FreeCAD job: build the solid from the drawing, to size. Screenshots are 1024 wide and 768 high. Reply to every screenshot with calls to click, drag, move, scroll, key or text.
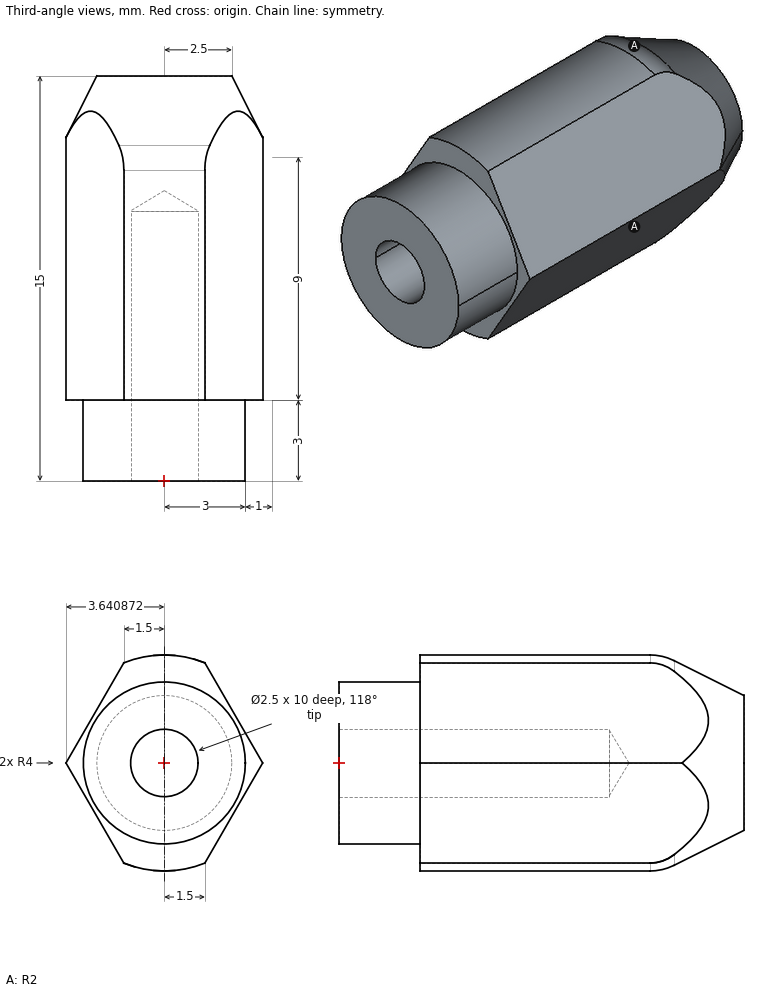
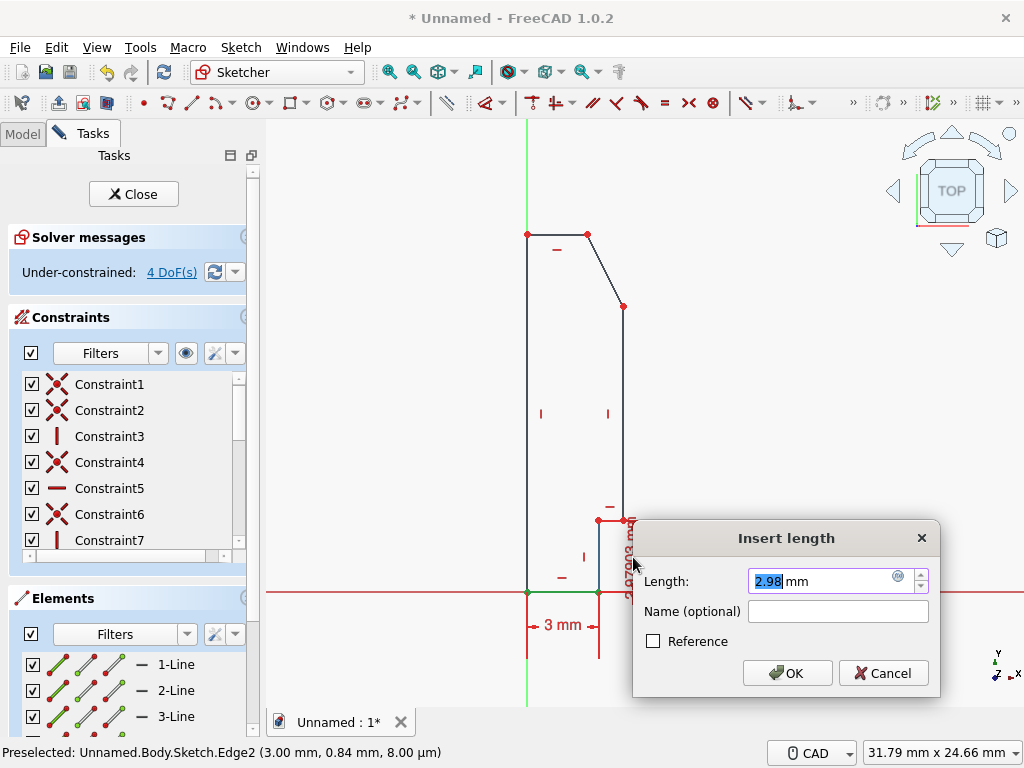
text(3)
key(Return)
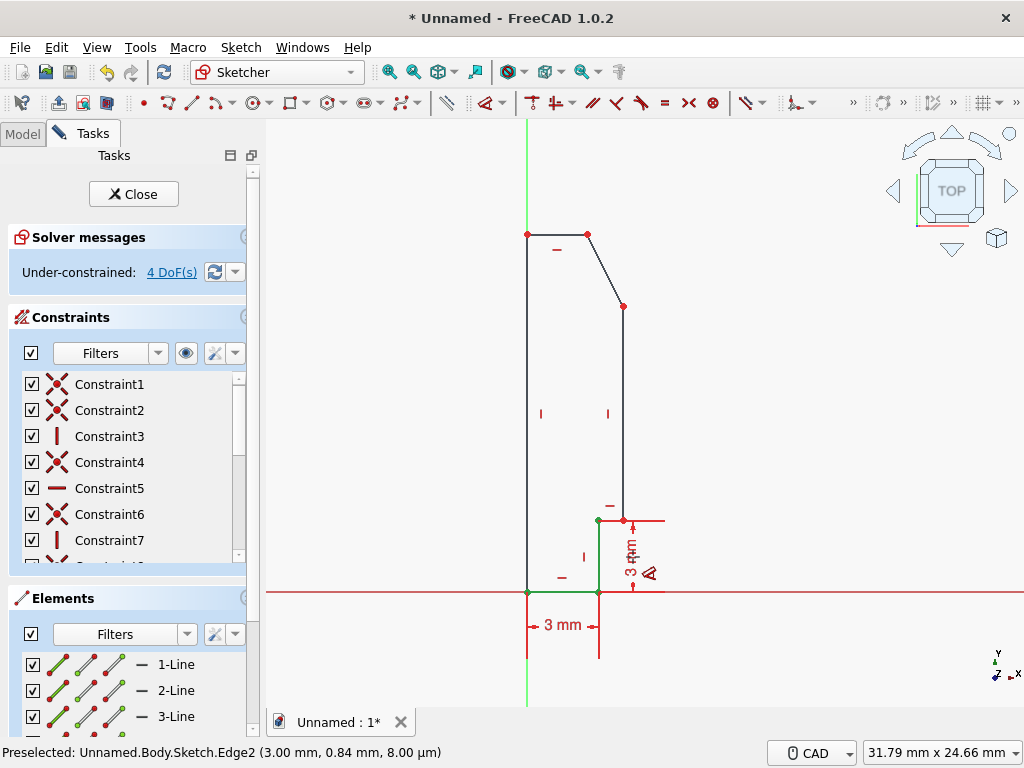
scroll(608, 520, up, 3)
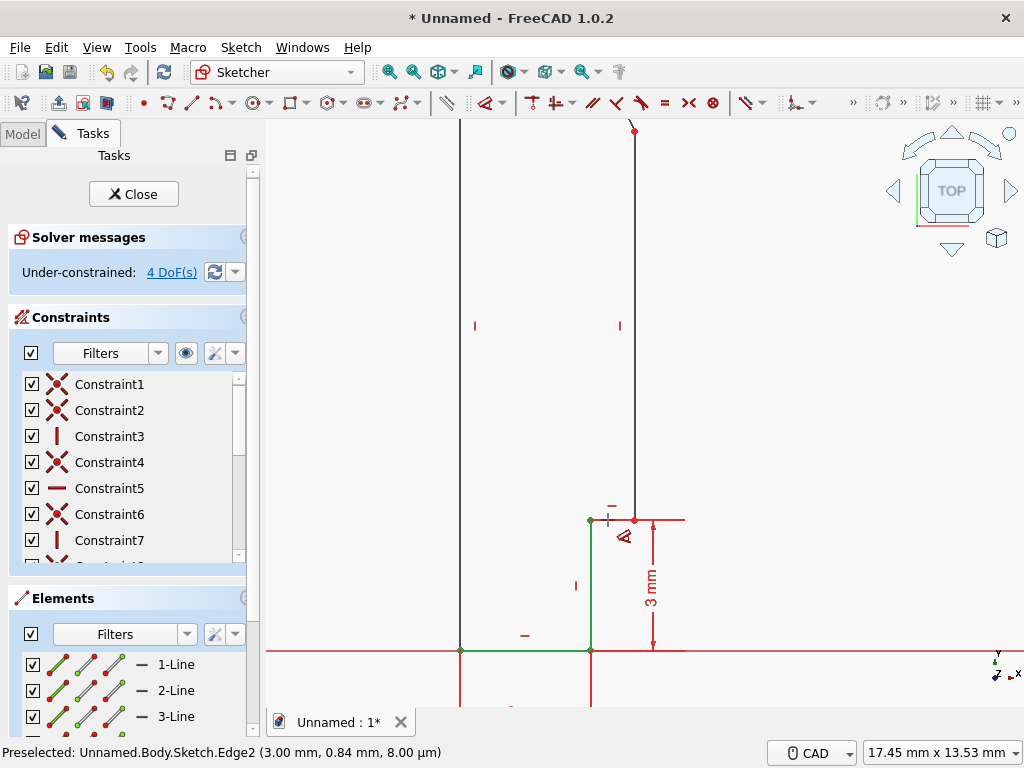
click(608, 520)
click(613, 554)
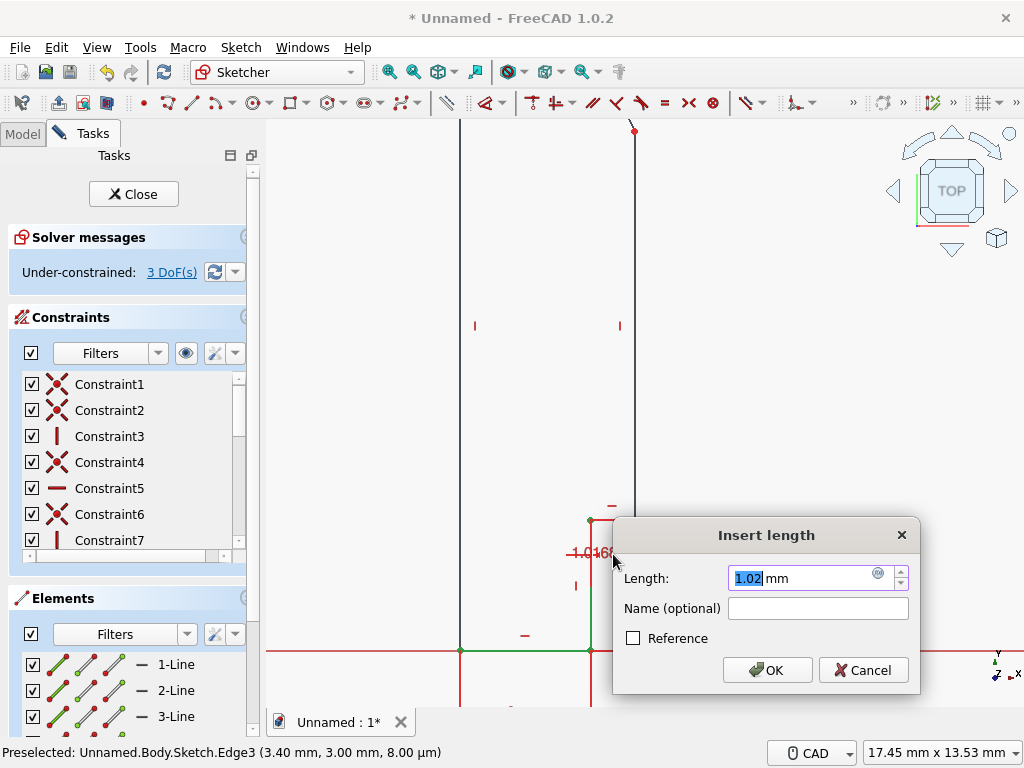
text(1)
key(Return)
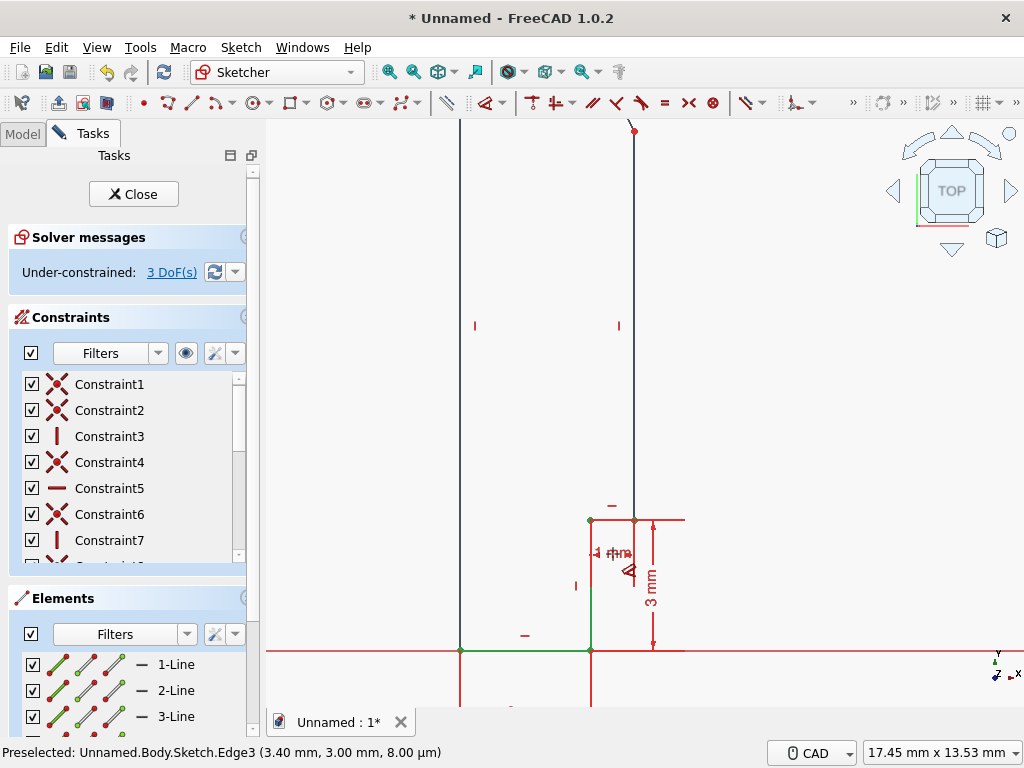
click(634, 404)
click(668, 334)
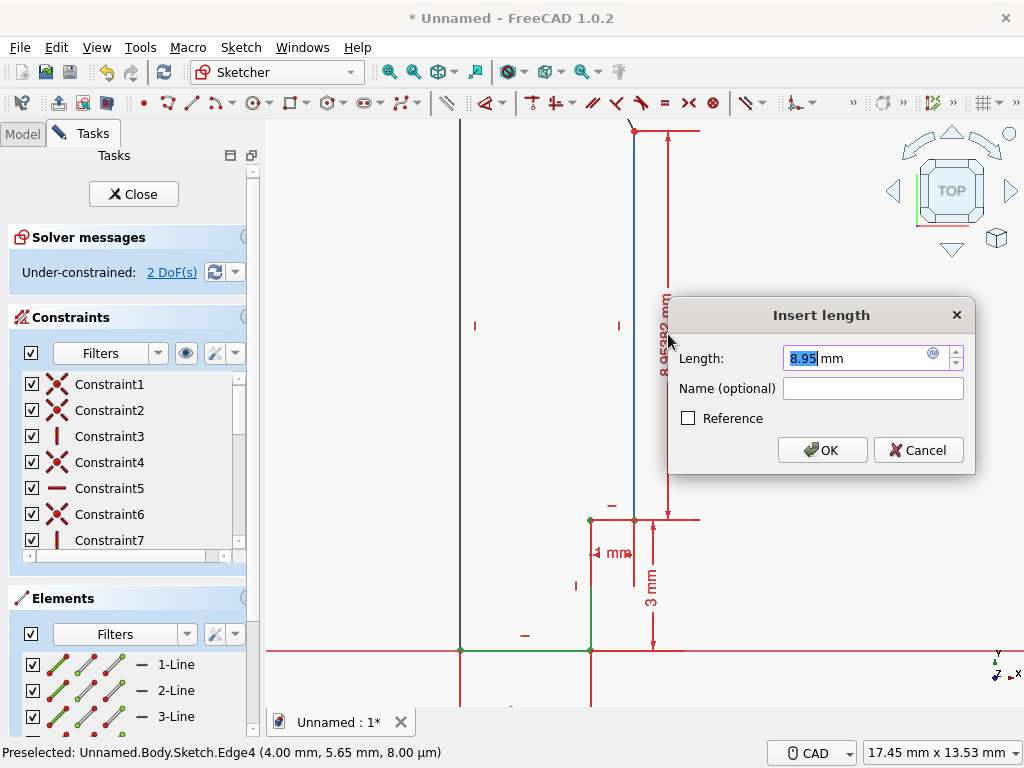
text(9)
key(Return)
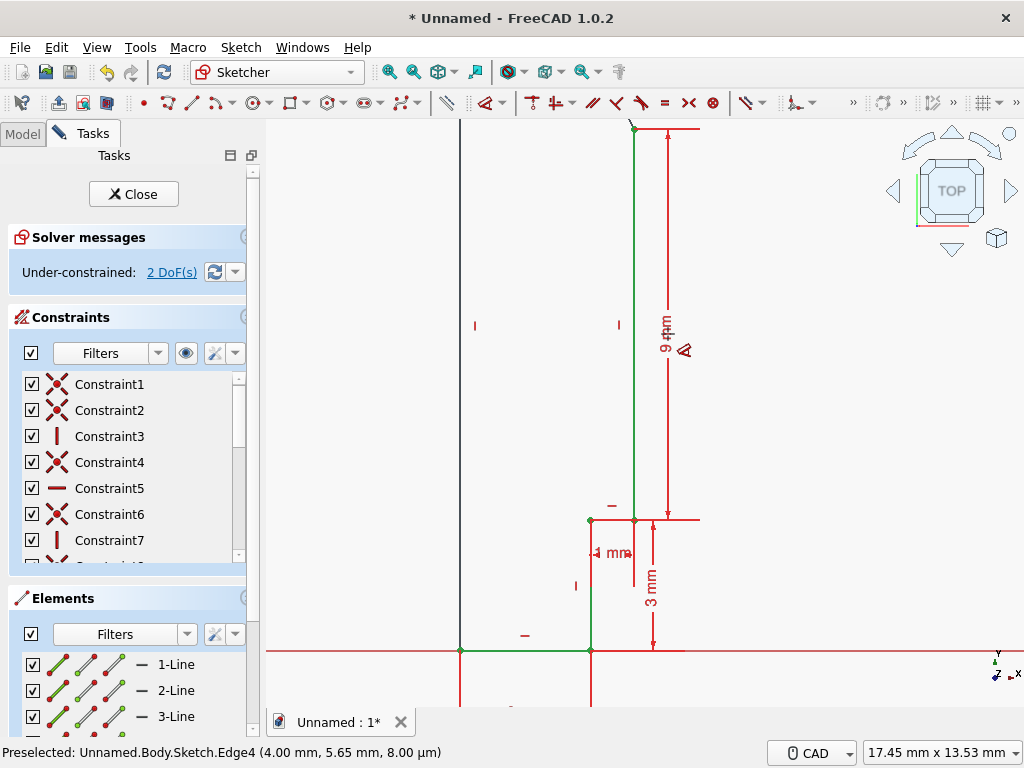
click(460, 195)
click(426, 399)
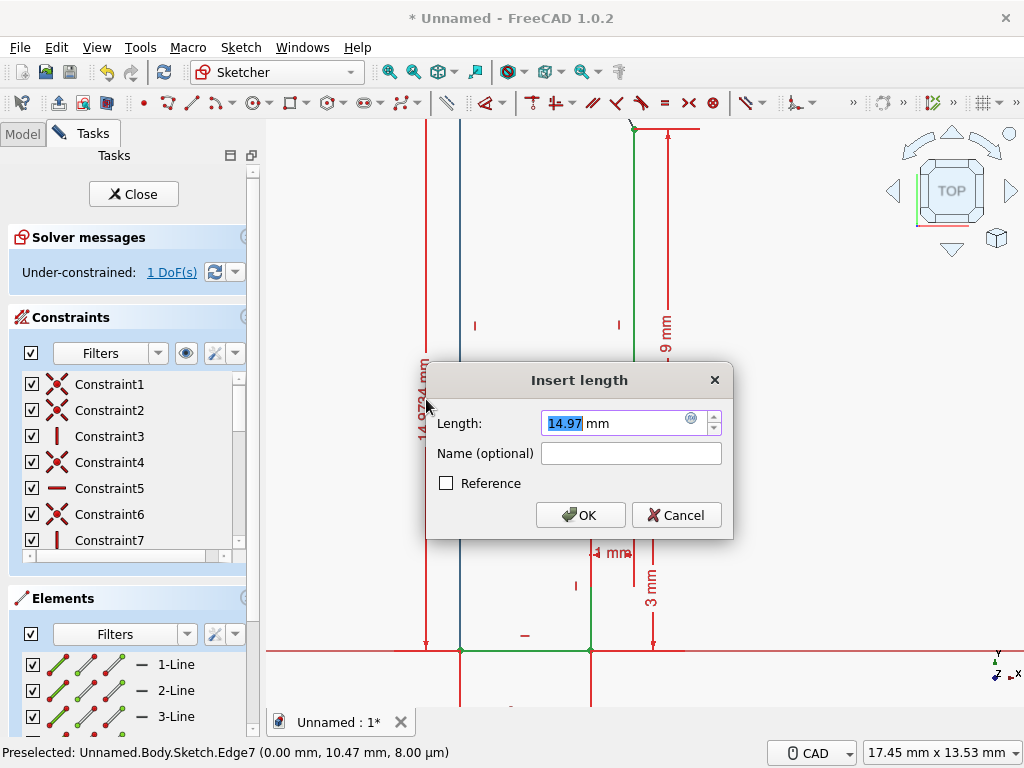
text(15)
key(Return)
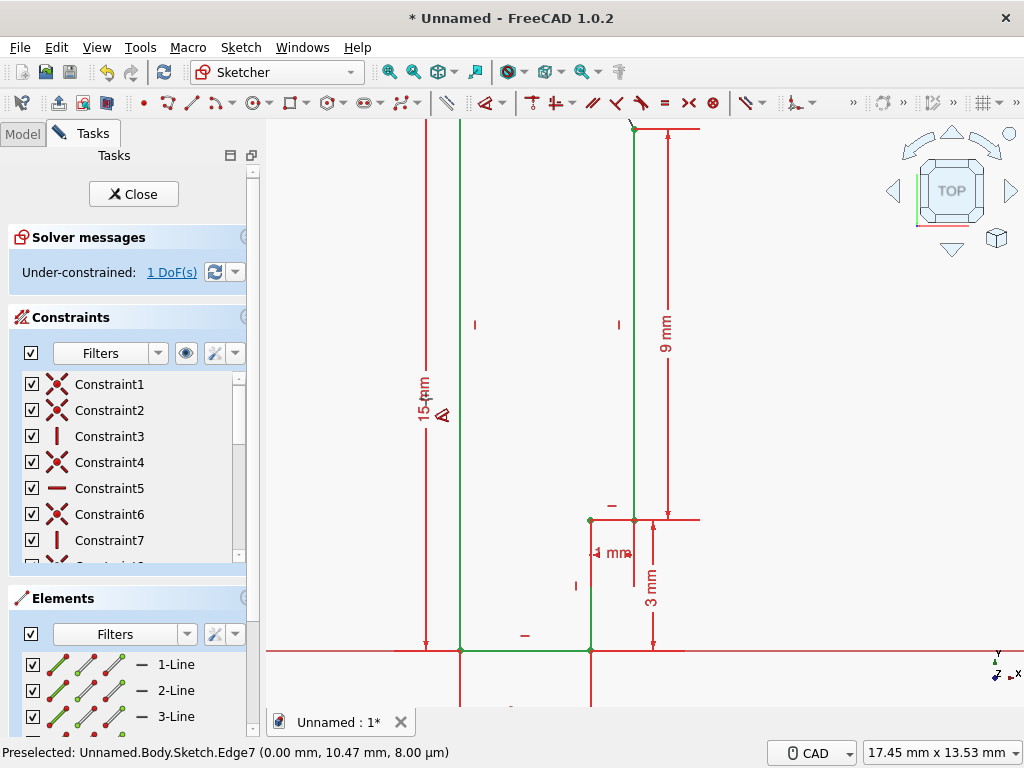
scroll(612, 520, down, 3)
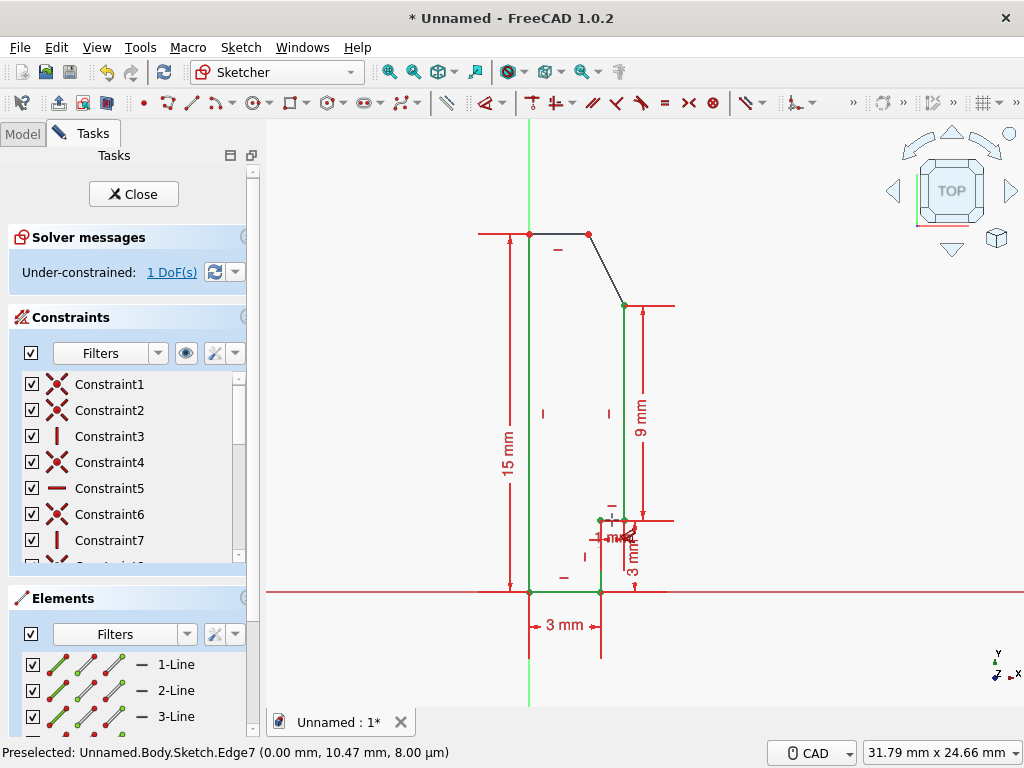
click(571, 234)
click(559, 200)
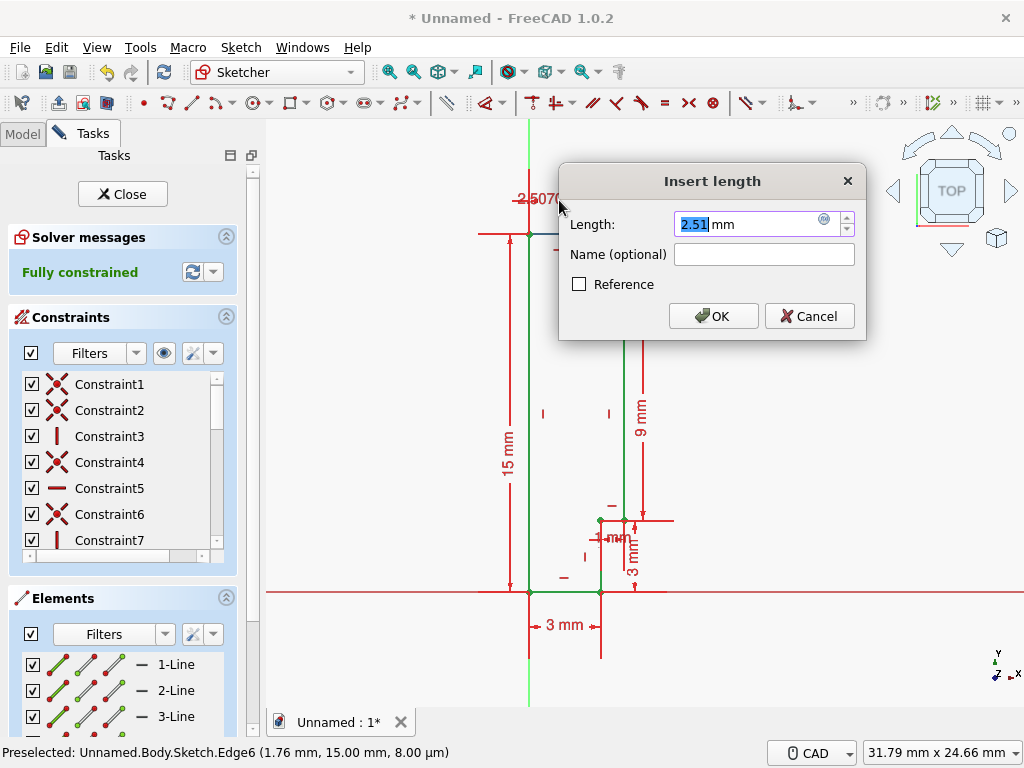
text(2.5)
key(Return)
key(Escape)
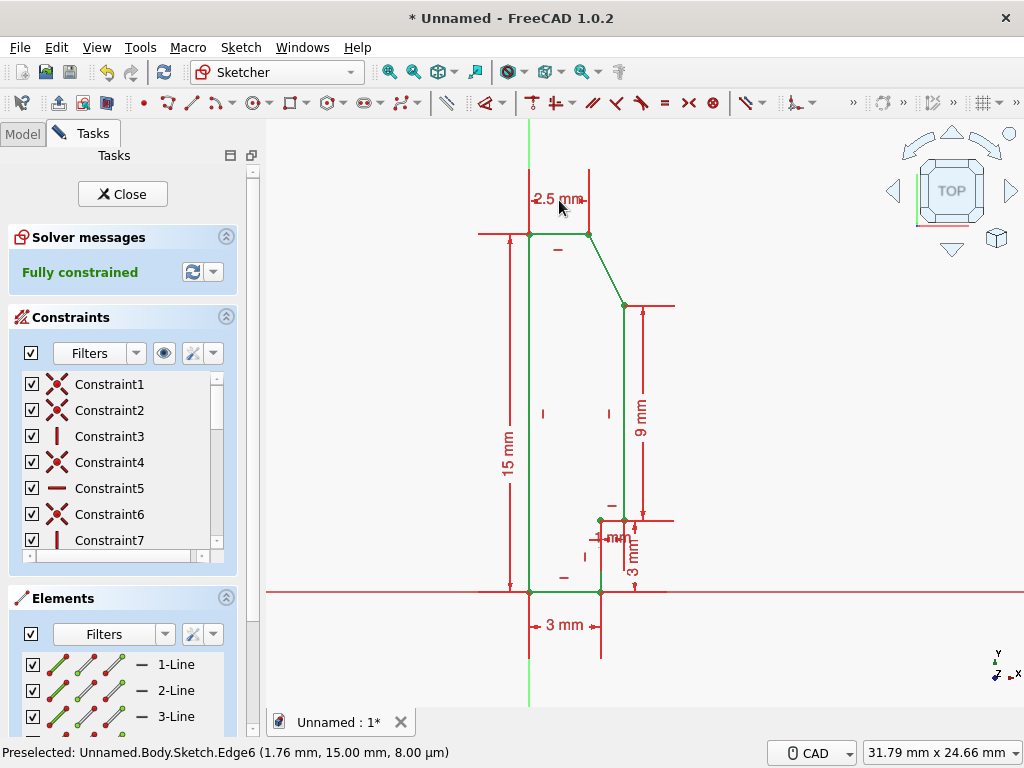
click(123, 194)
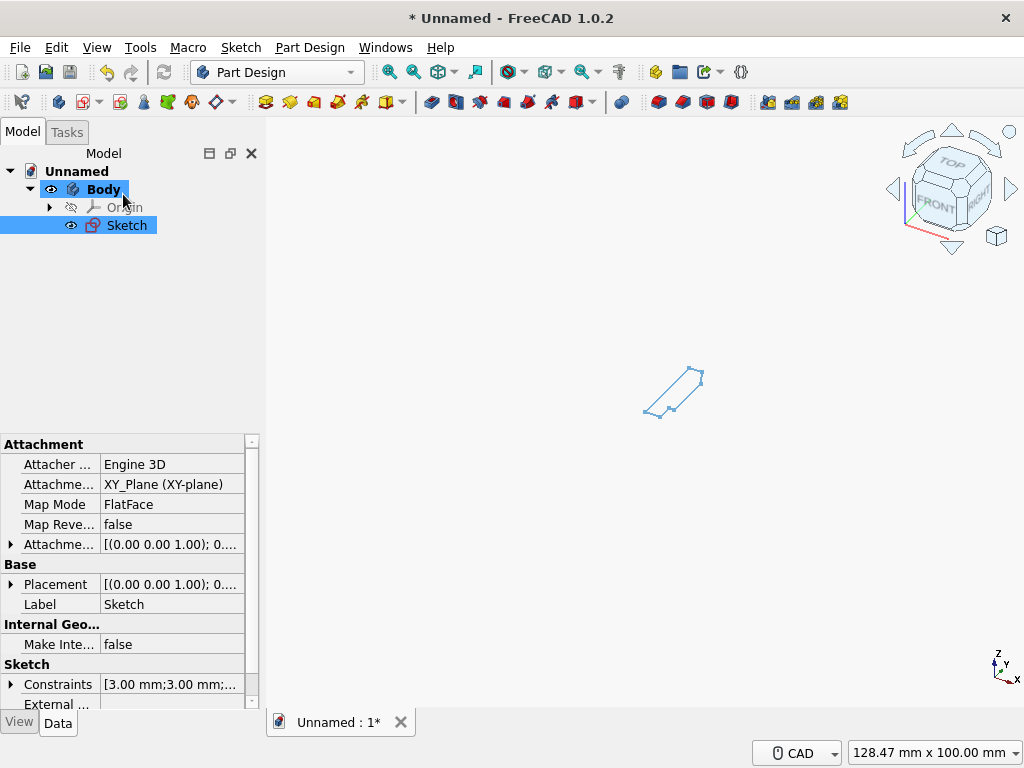
click(290, 102)